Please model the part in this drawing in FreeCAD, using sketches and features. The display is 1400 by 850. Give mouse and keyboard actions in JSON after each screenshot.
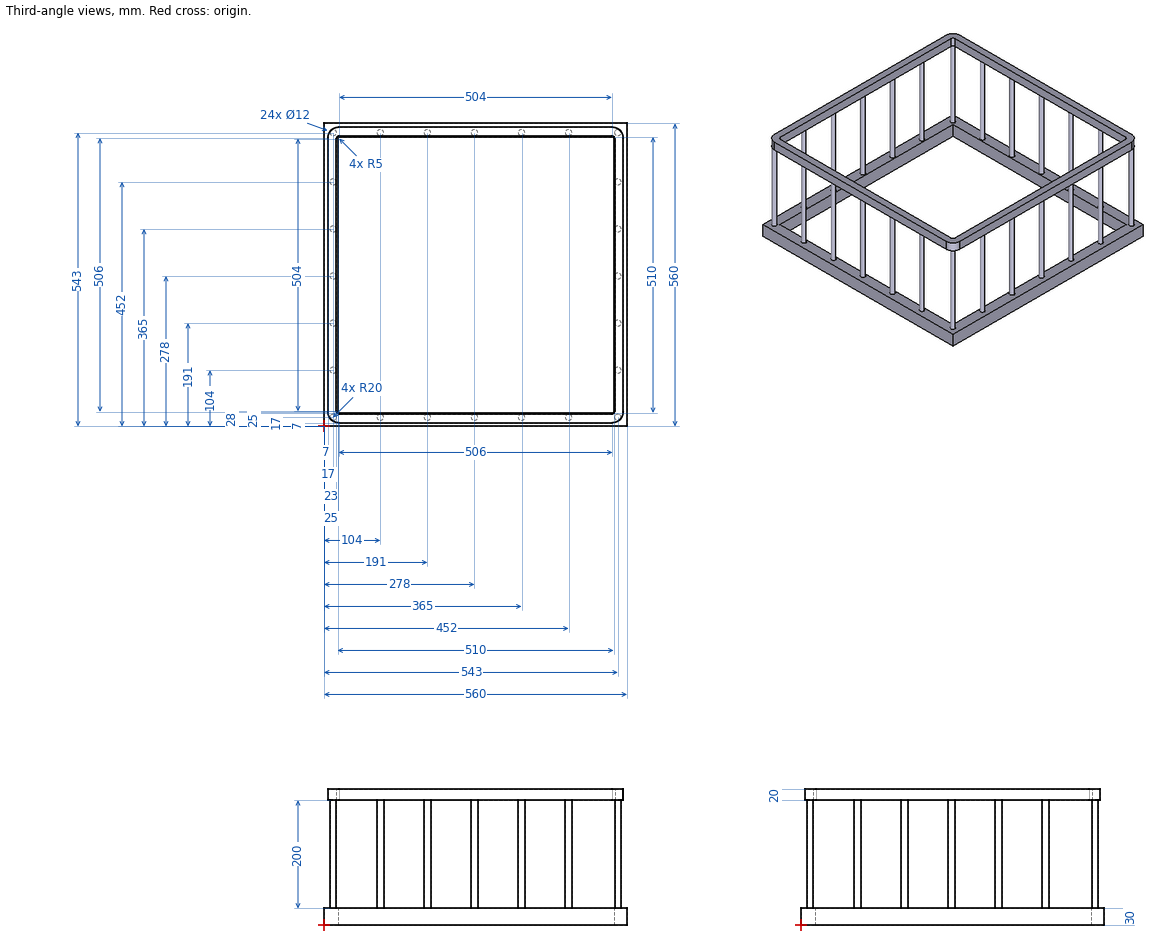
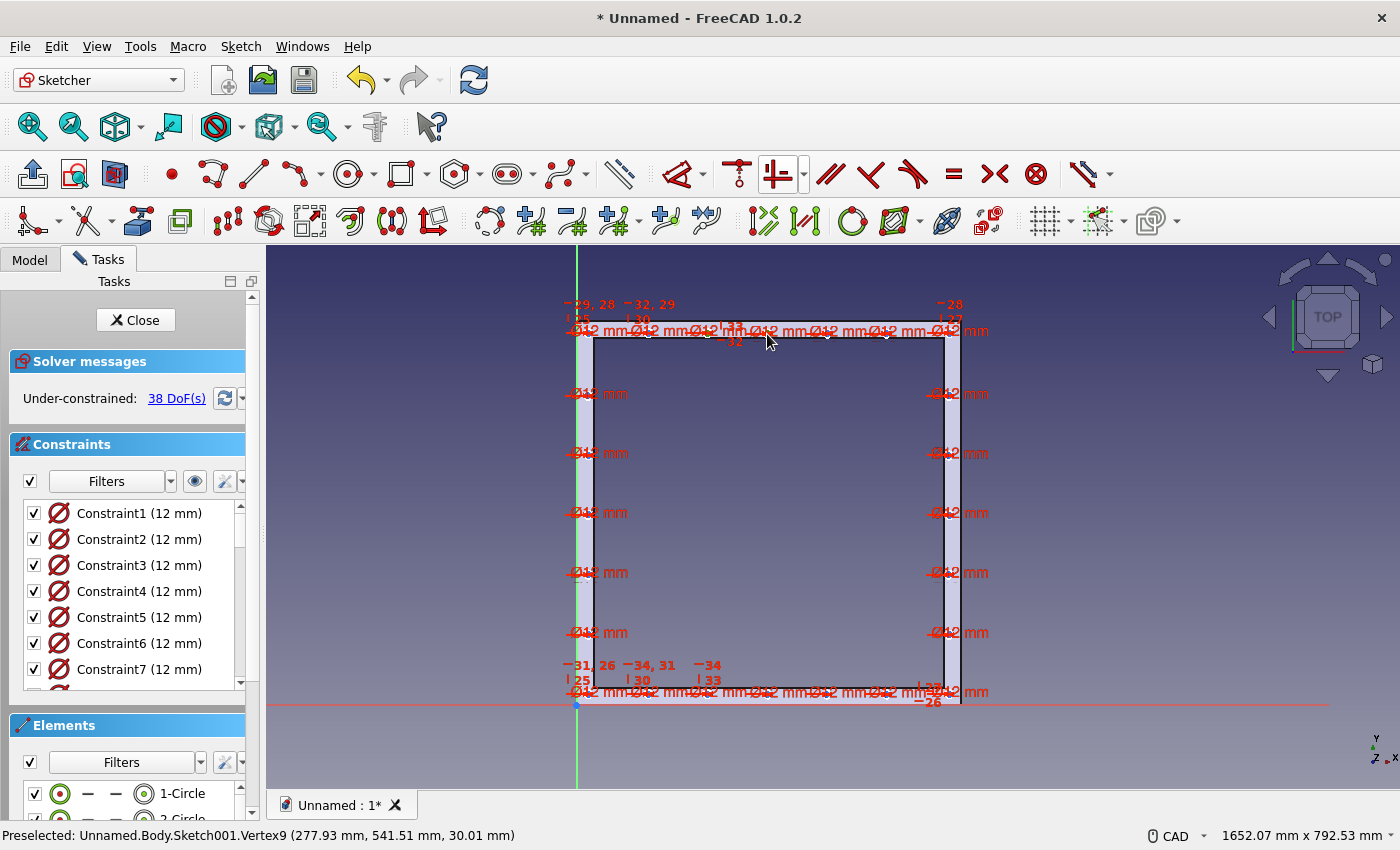
{"action": "left_click", "coordinate": [804, 174]}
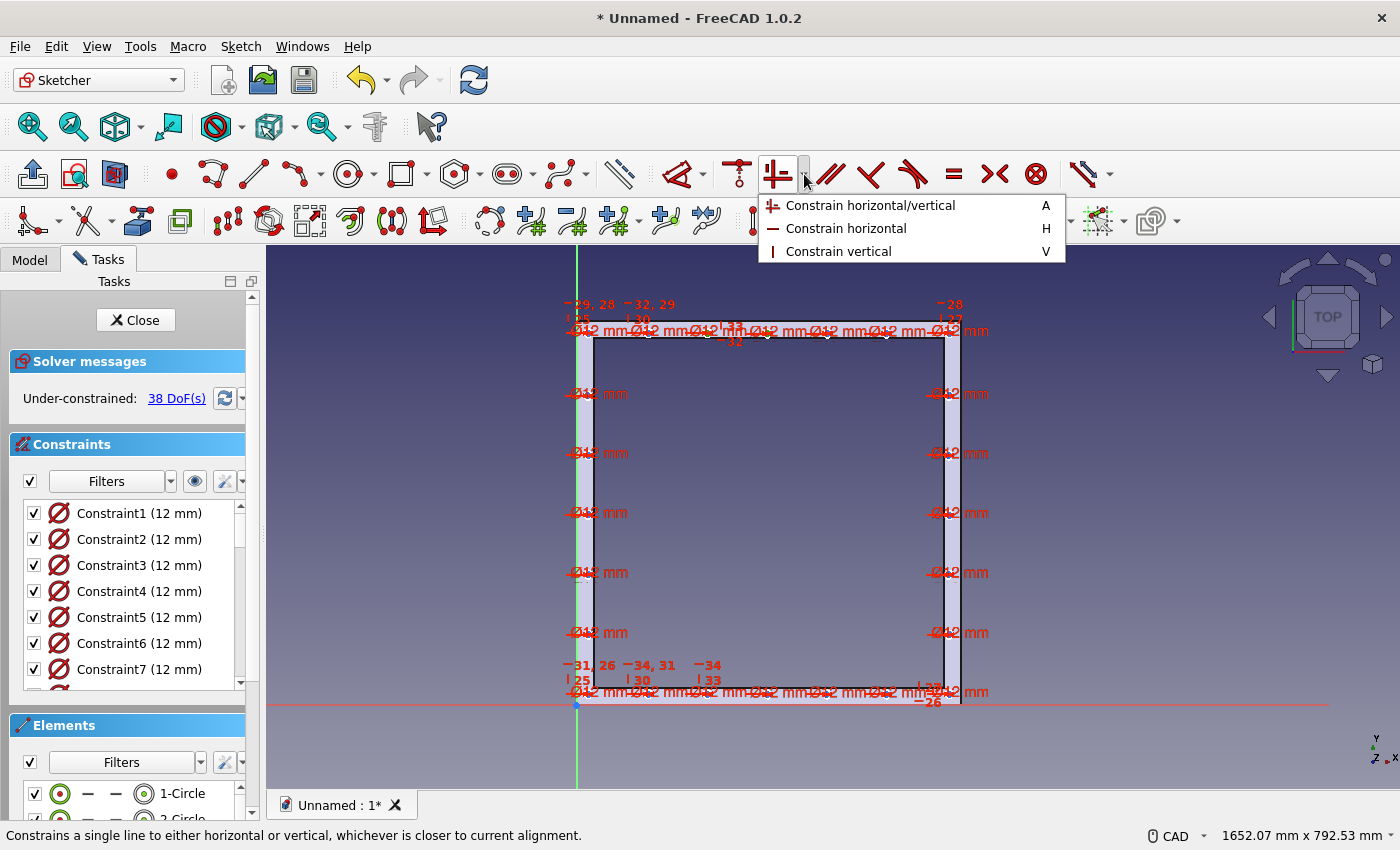
{"action": "left_click", "coordinate": [912, 228]}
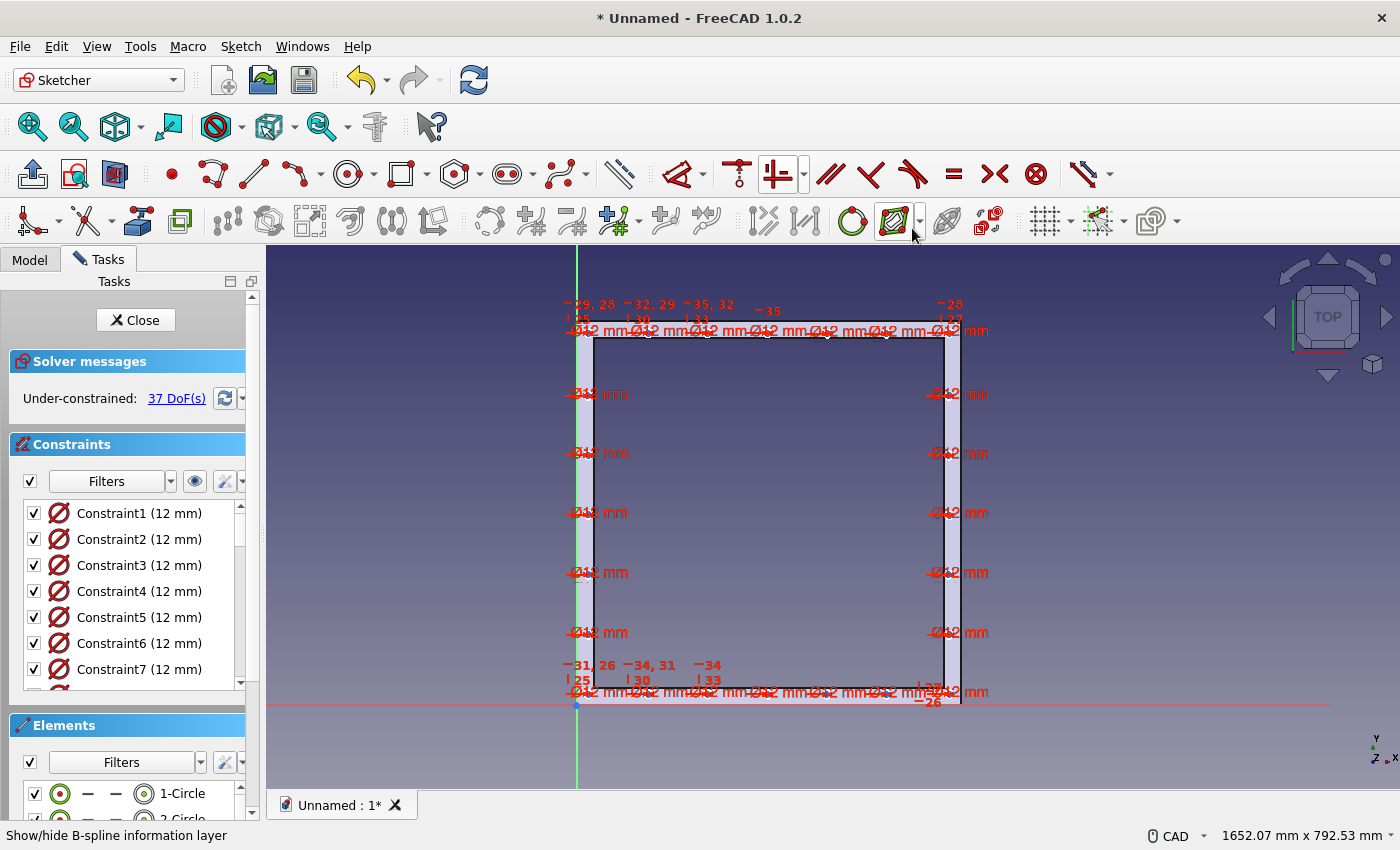
{"action": "left_click", "coordinate": [767, 333]}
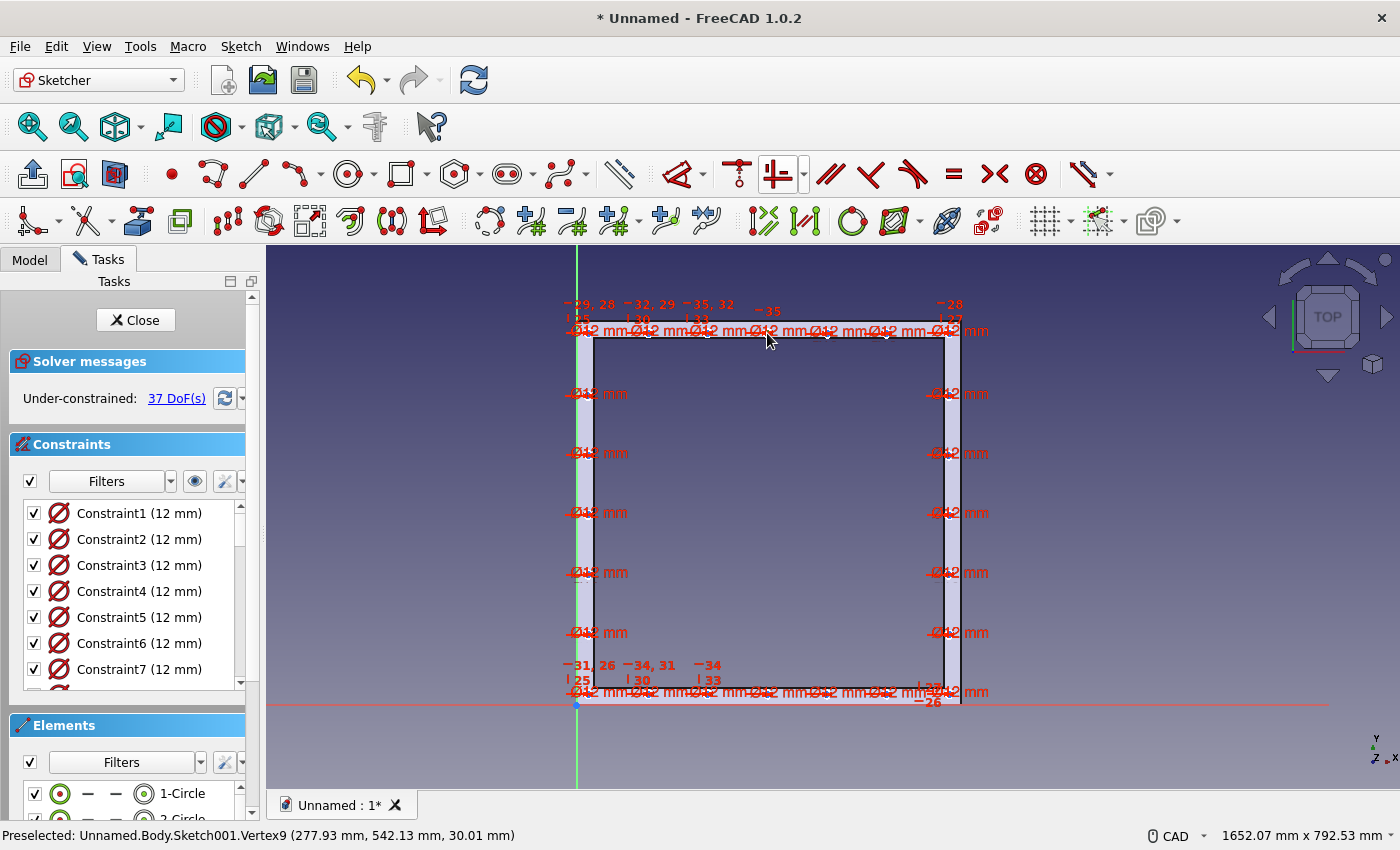
{"action": "left_click", "coordinate": [768, 694]}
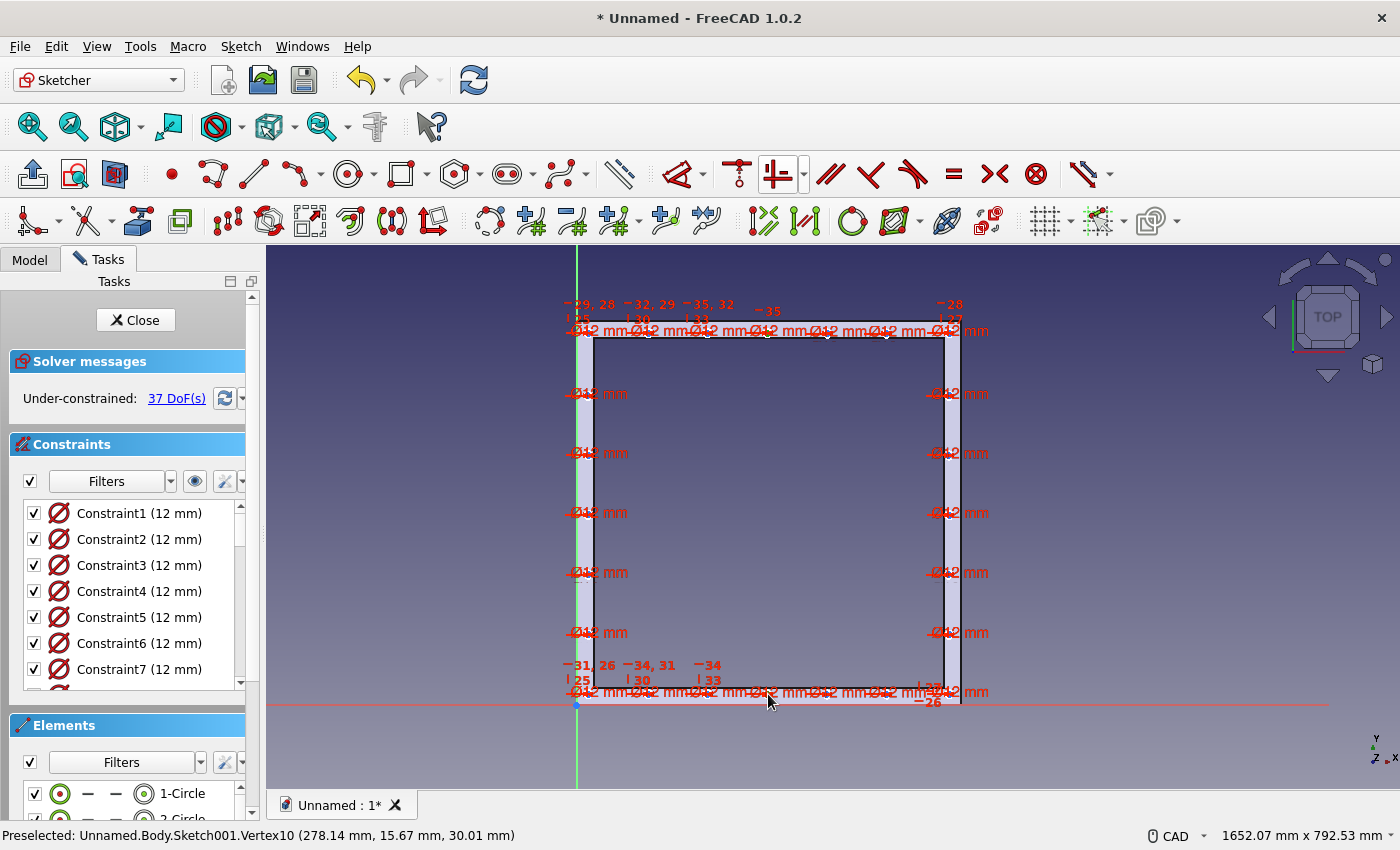
{"action": "key", "text": "v"}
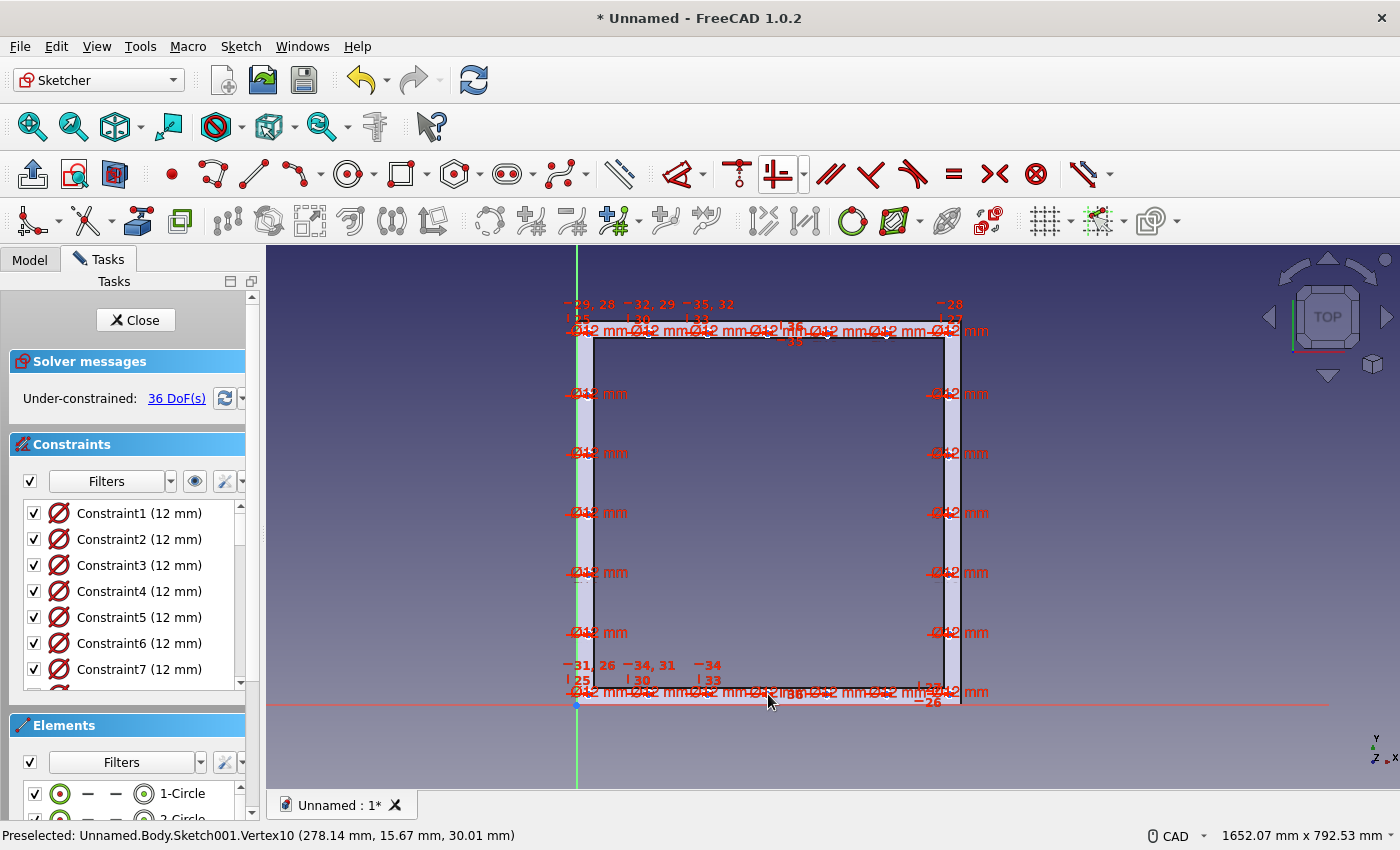
{"action": "left_click", "coordinate": [707, 694]}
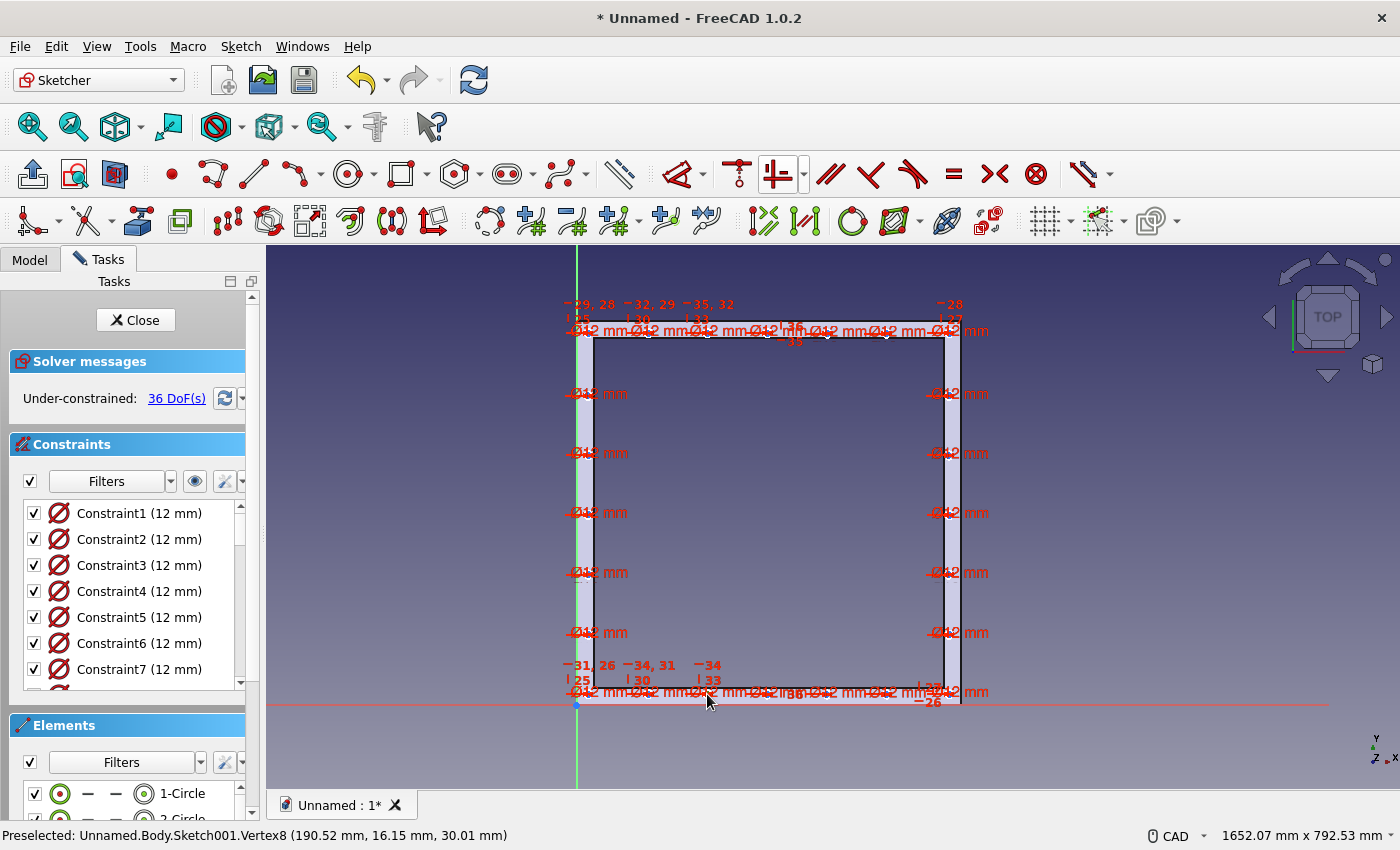
{"action": "left_click", "coordinate": [767, 694]}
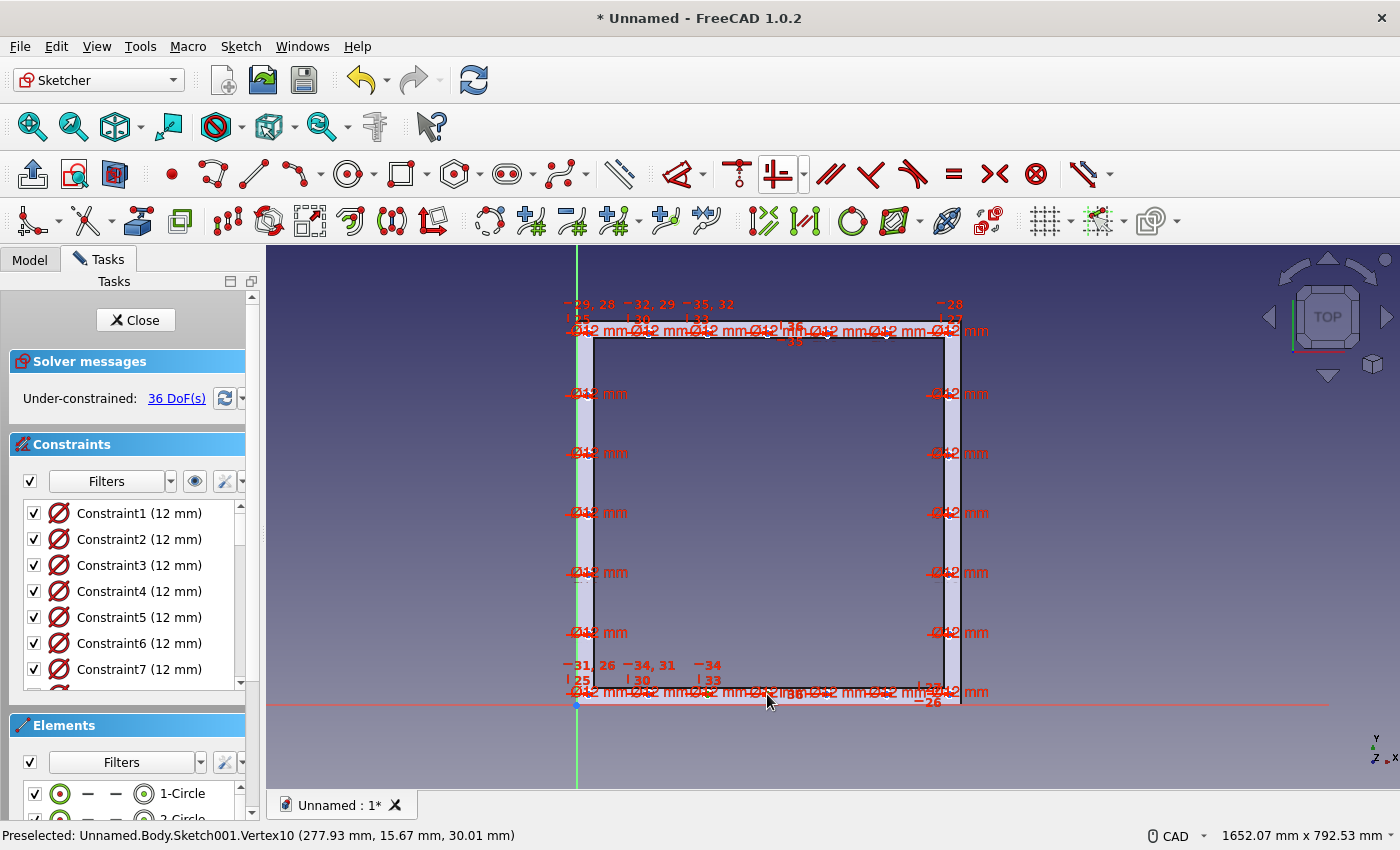
{"action": "key", "text": "h"}